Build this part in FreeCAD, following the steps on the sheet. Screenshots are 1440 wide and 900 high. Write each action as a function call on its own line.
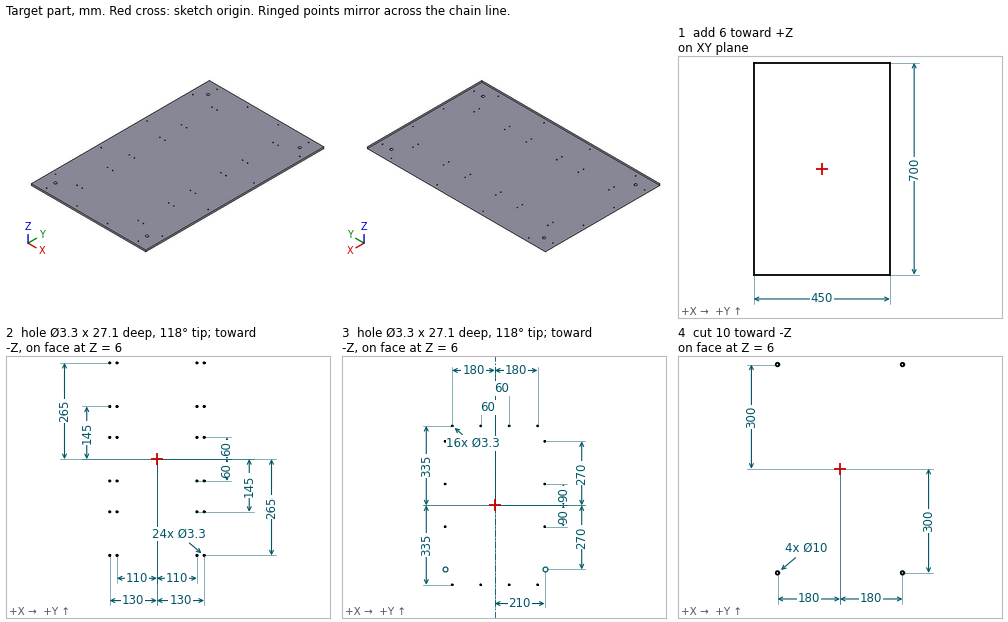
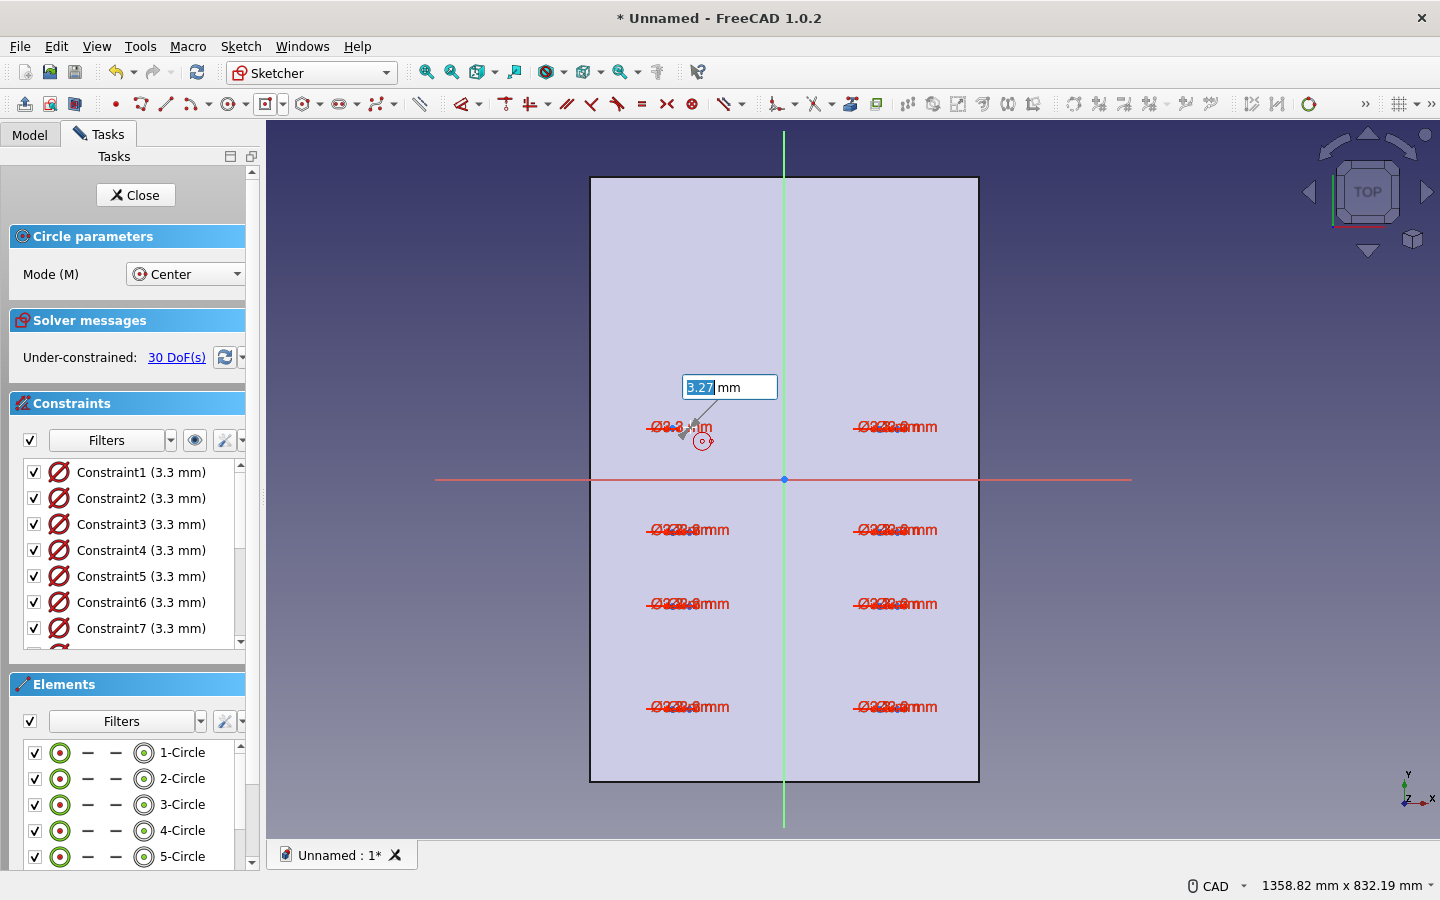
text(3.3)
key(Return)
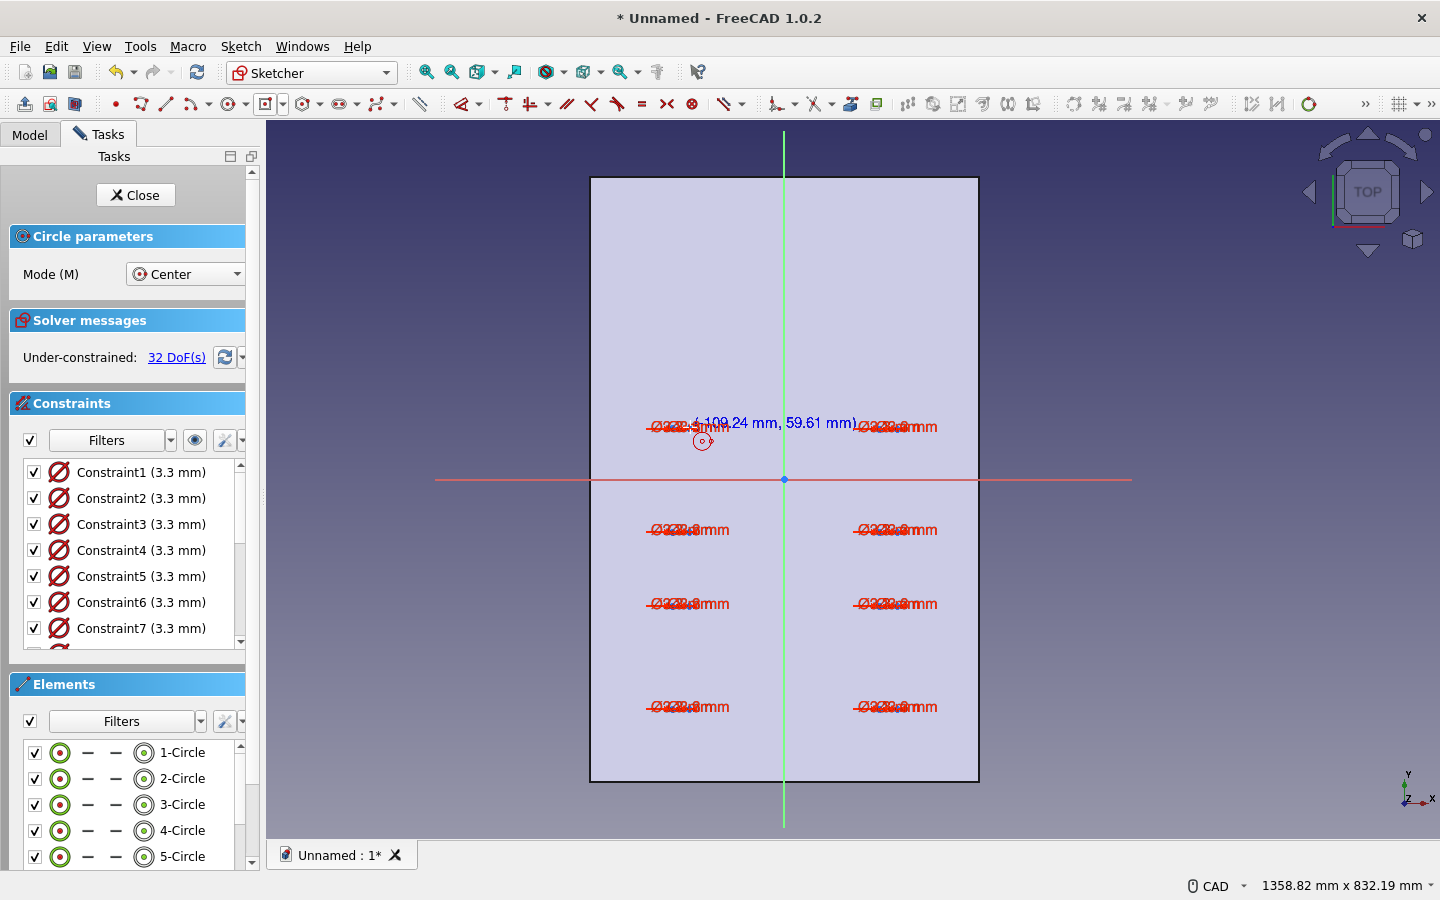
scroll(672, 354, up, 14)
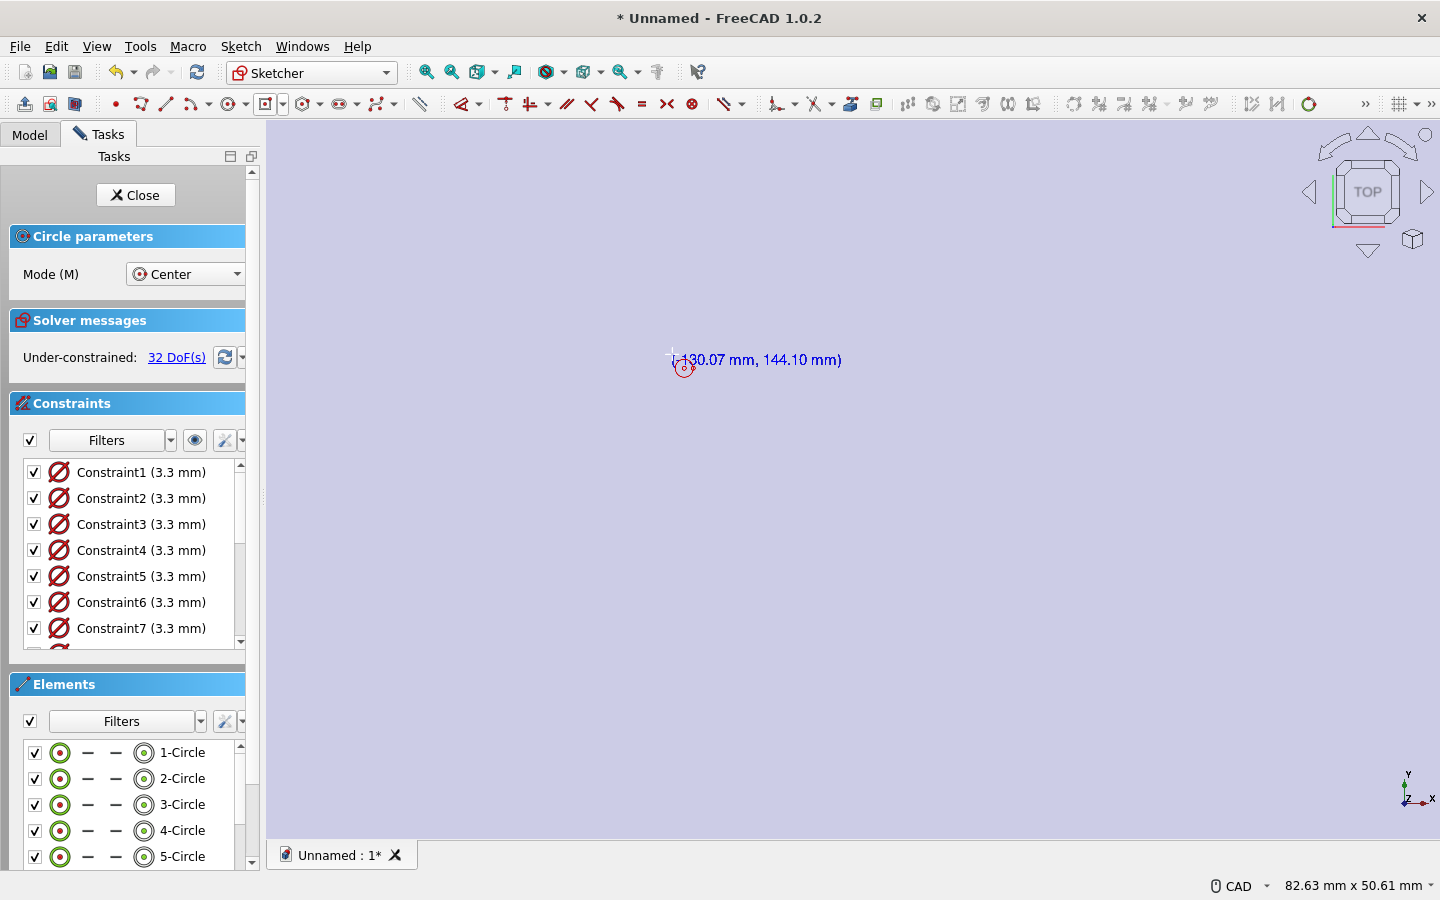
scroll(672, 354, down, 14)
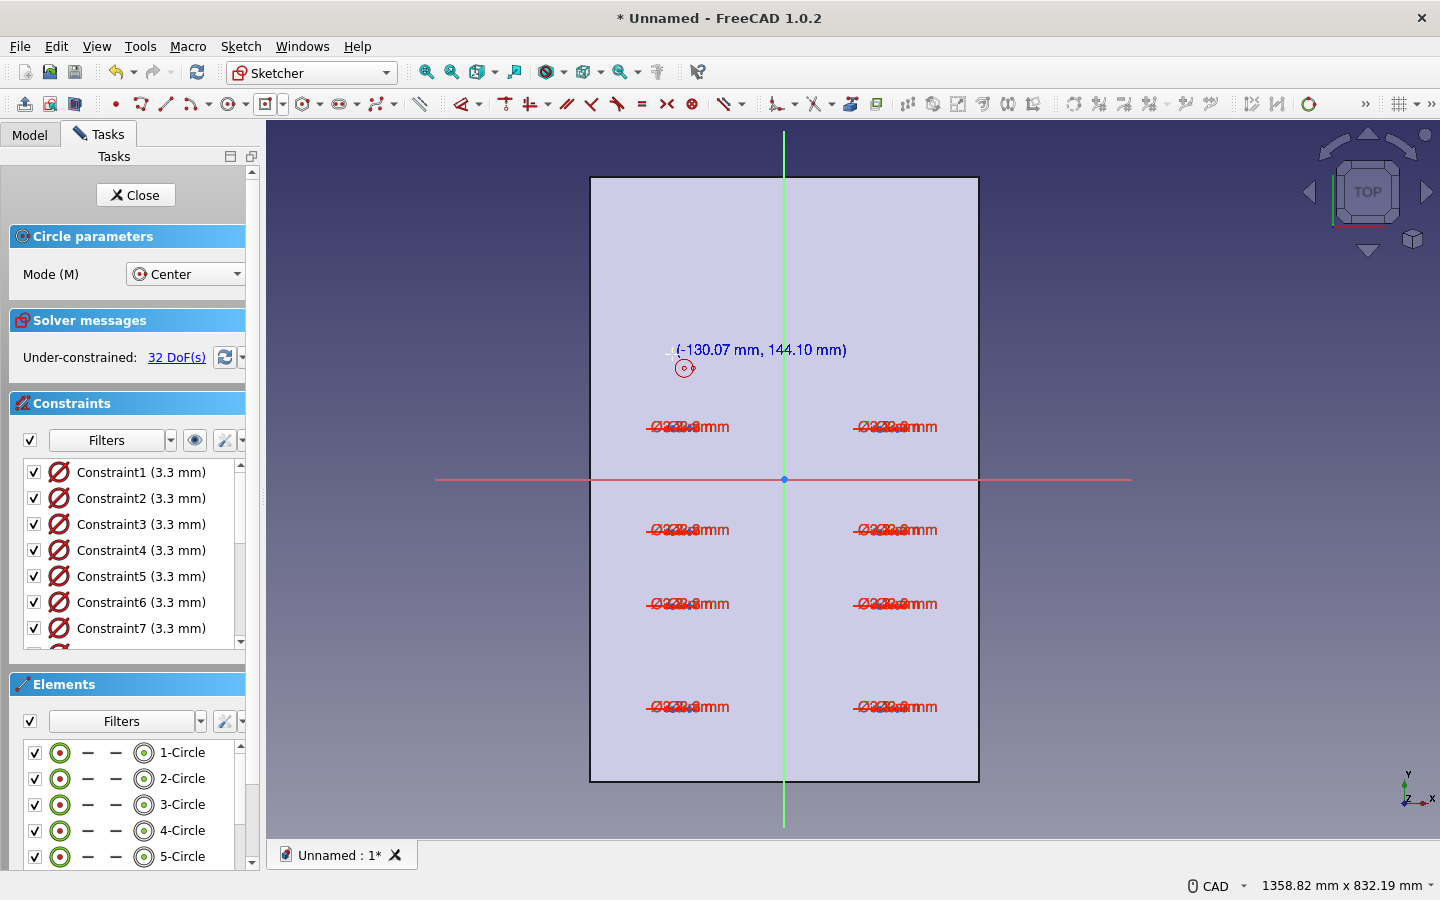
click(672, 354)
move(673, 353)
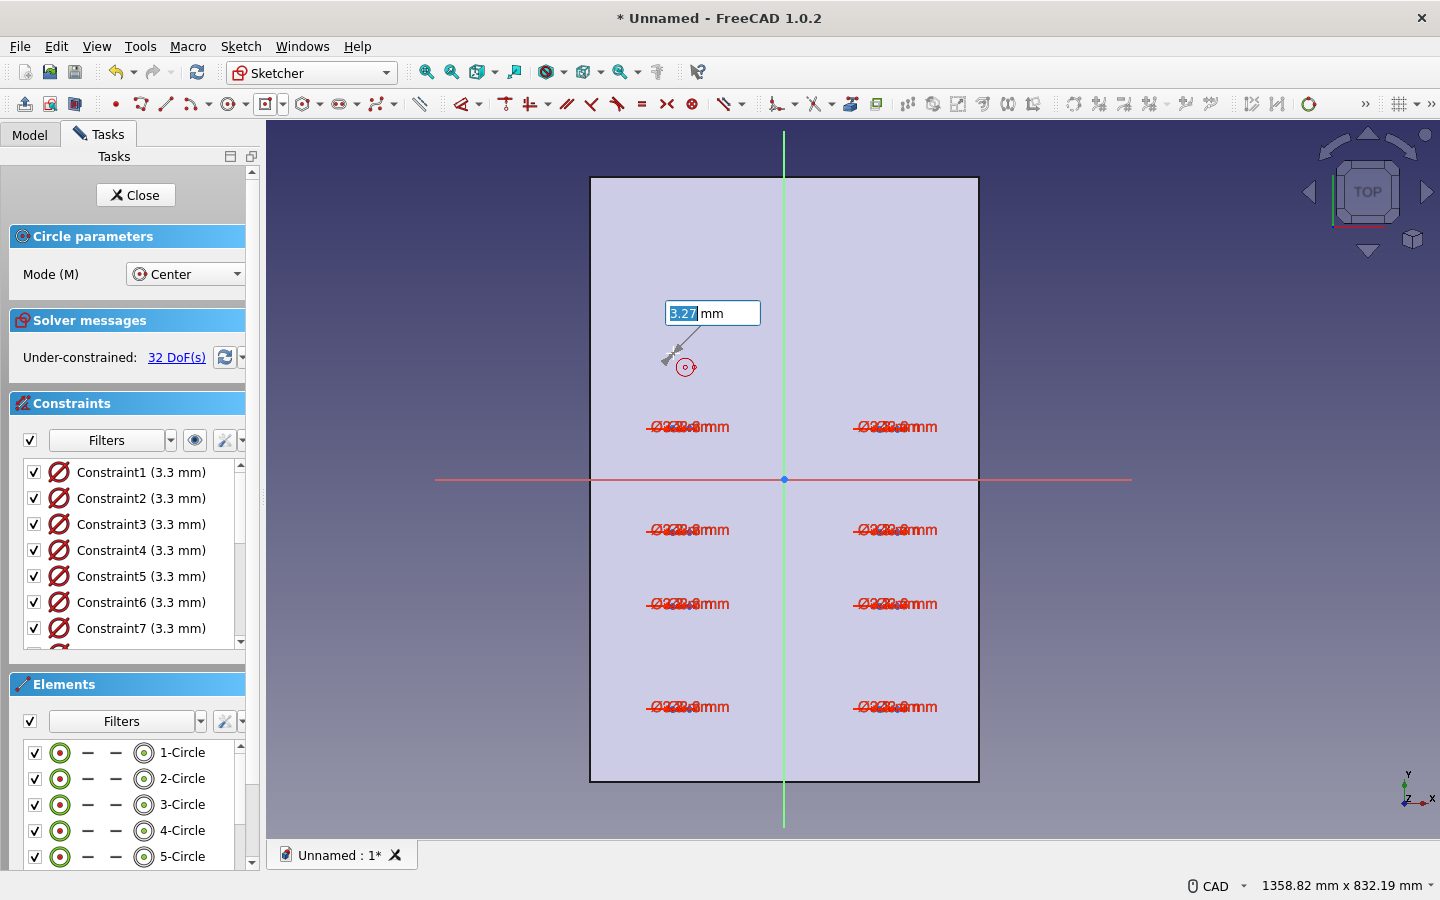
text(3.3)
key(Return)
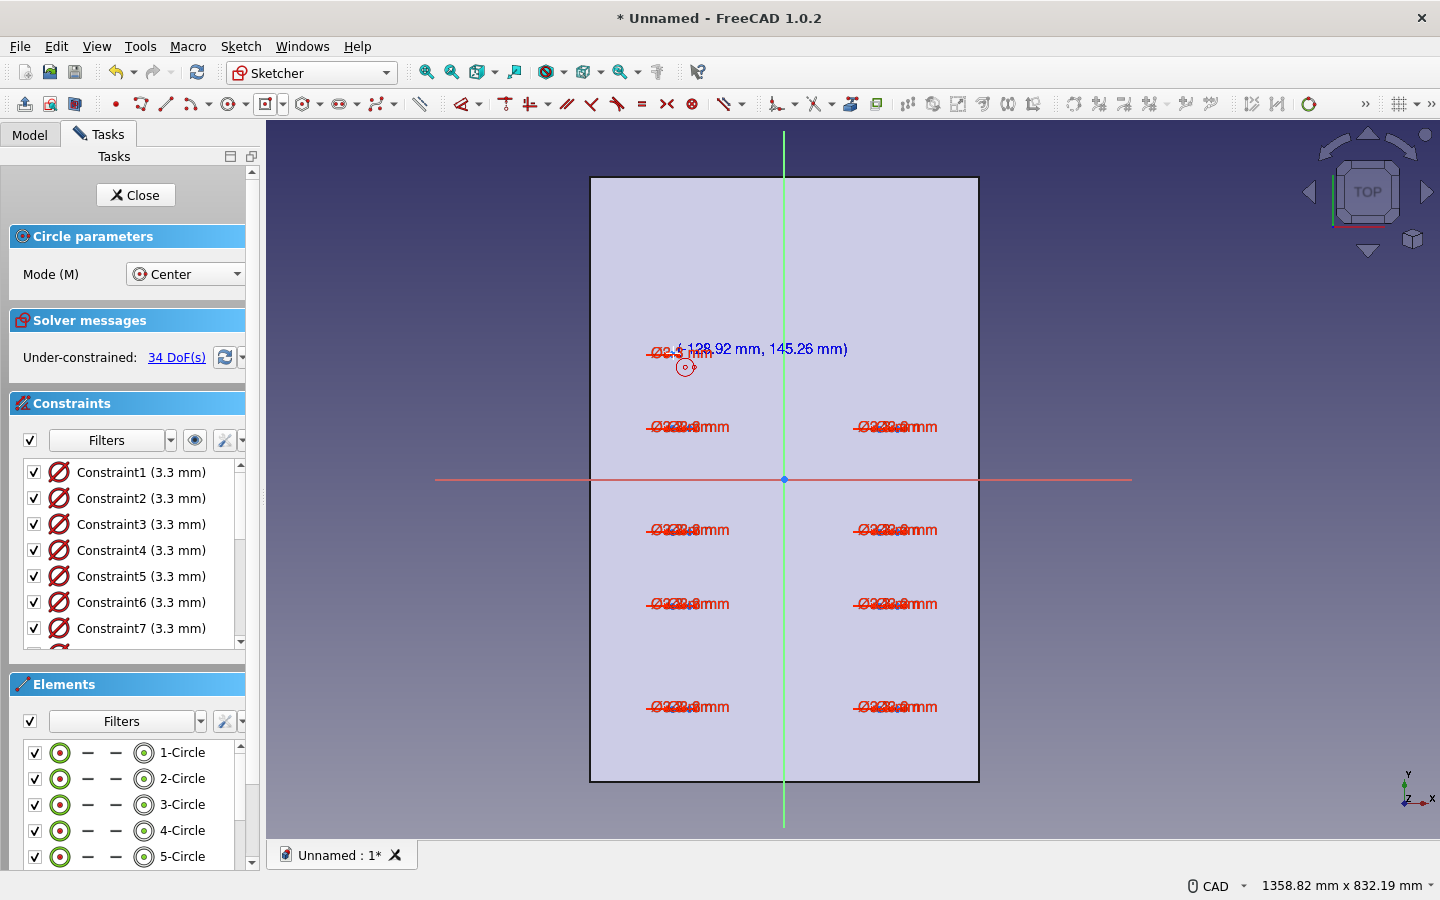
scroll(689, 354, up, 14)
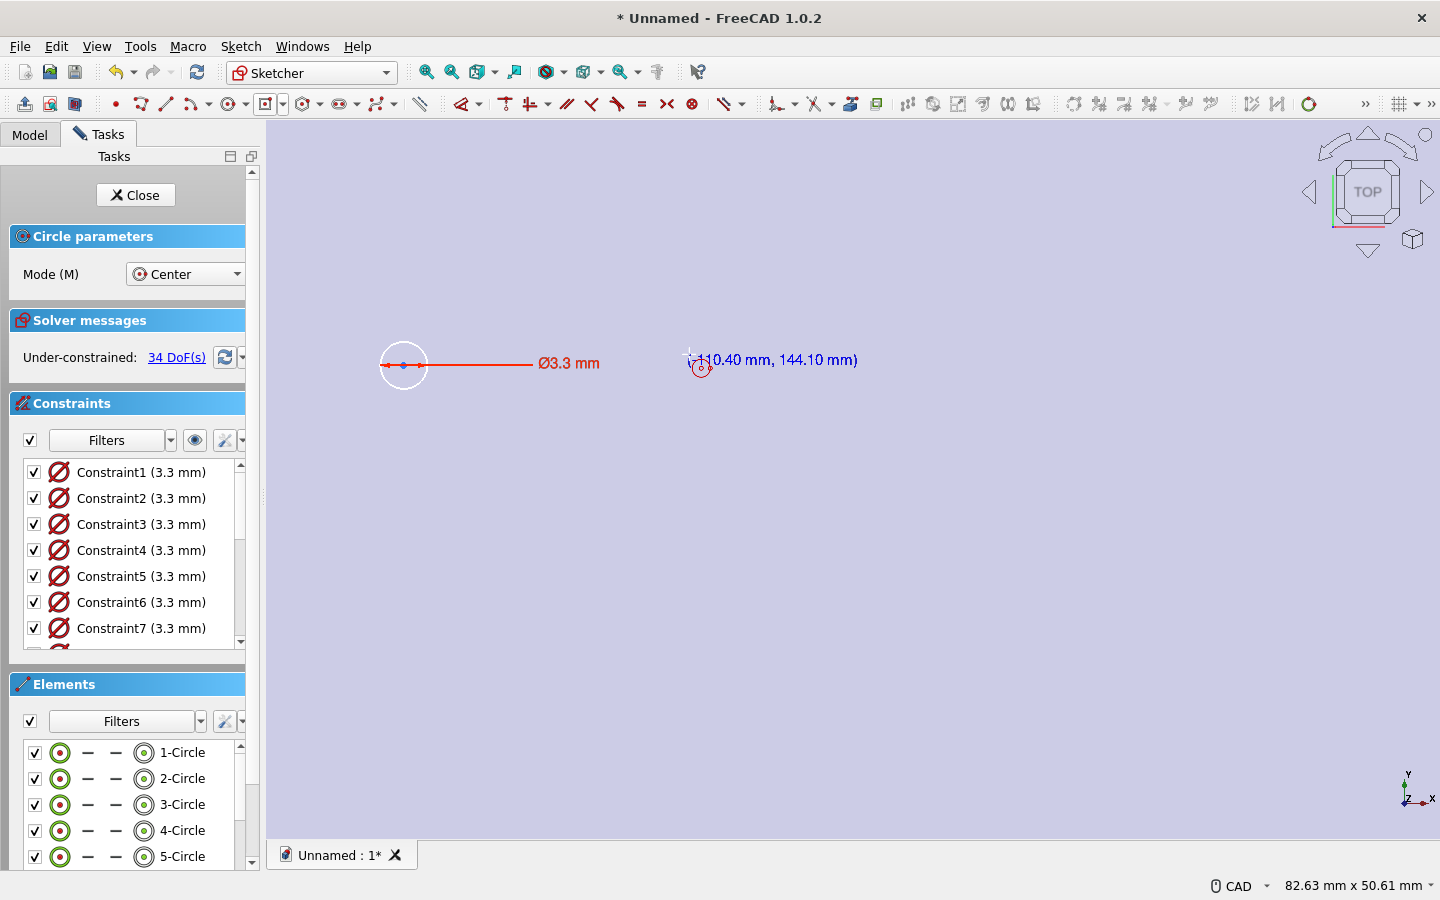
scroll(689, 354, down, 14)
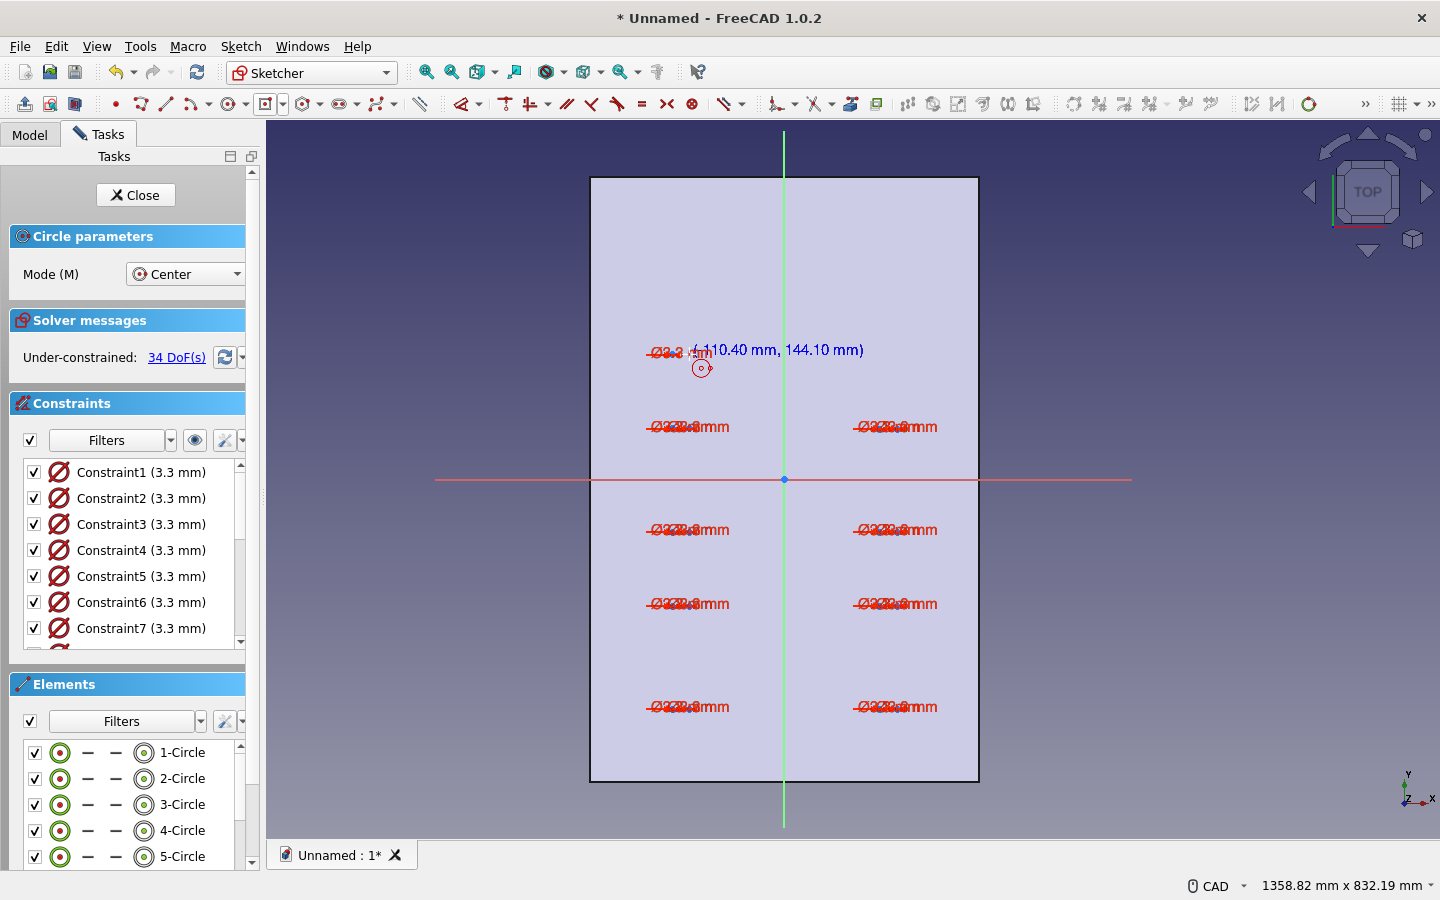
click(689, 354)
move(690, 353)